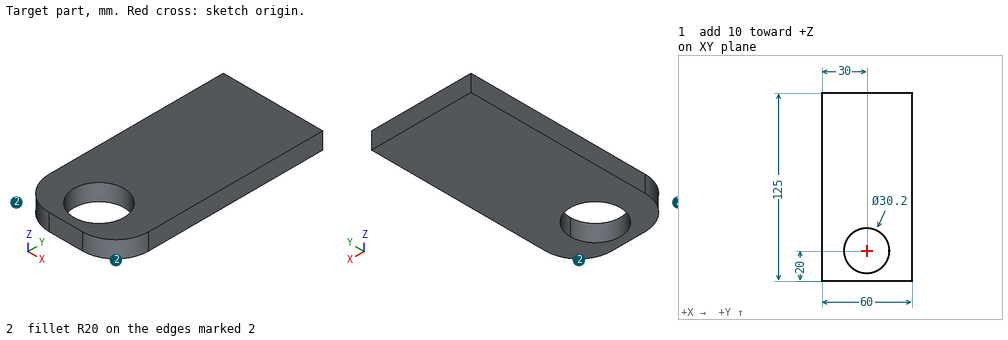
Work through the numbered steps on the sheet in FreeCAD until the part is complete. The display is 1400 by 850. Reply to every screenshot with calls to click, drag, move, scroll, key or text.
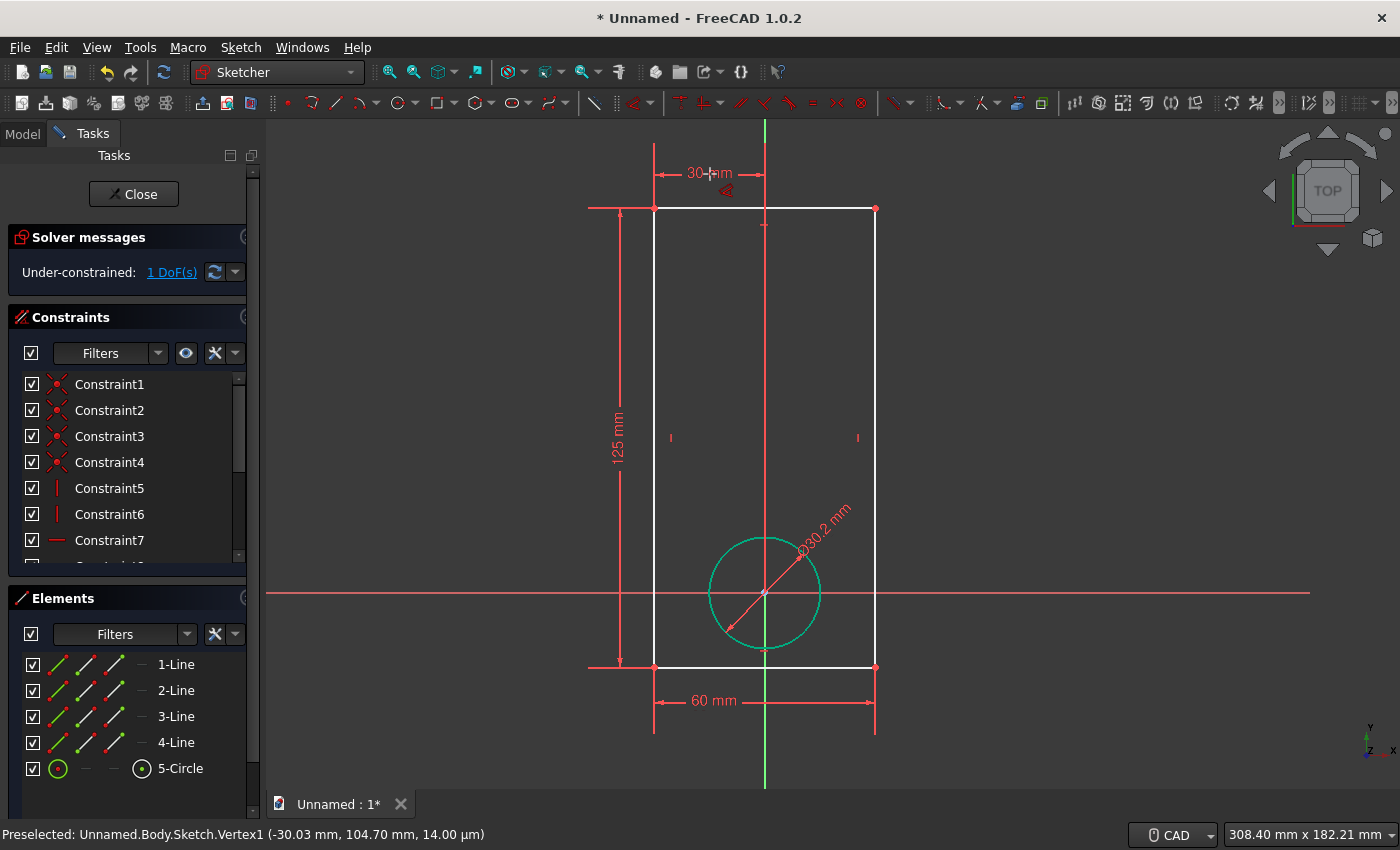
click(654, 668)
click(620, 630)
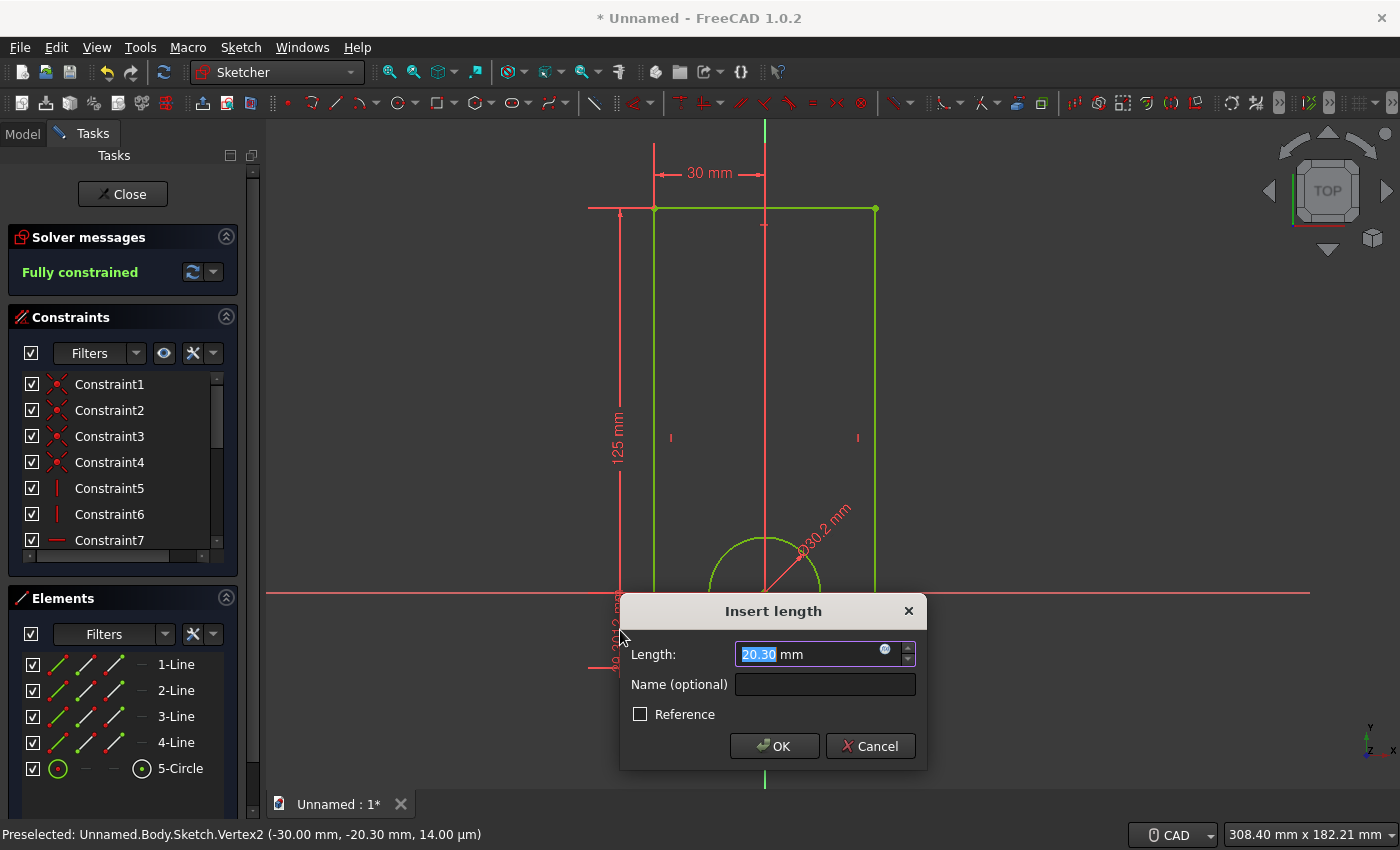
text(20)
key(Return)
key(Escape)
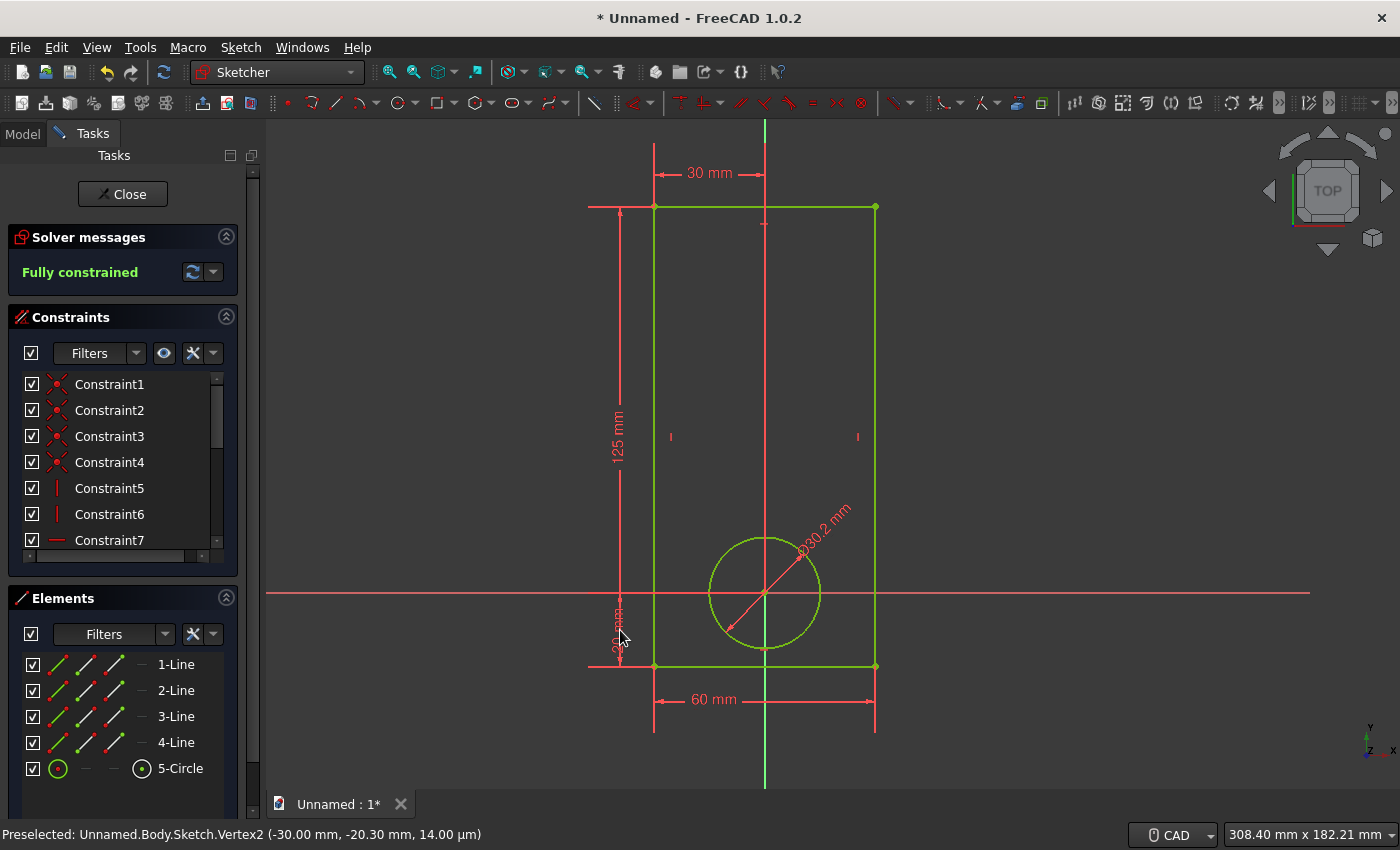
click(123, 194)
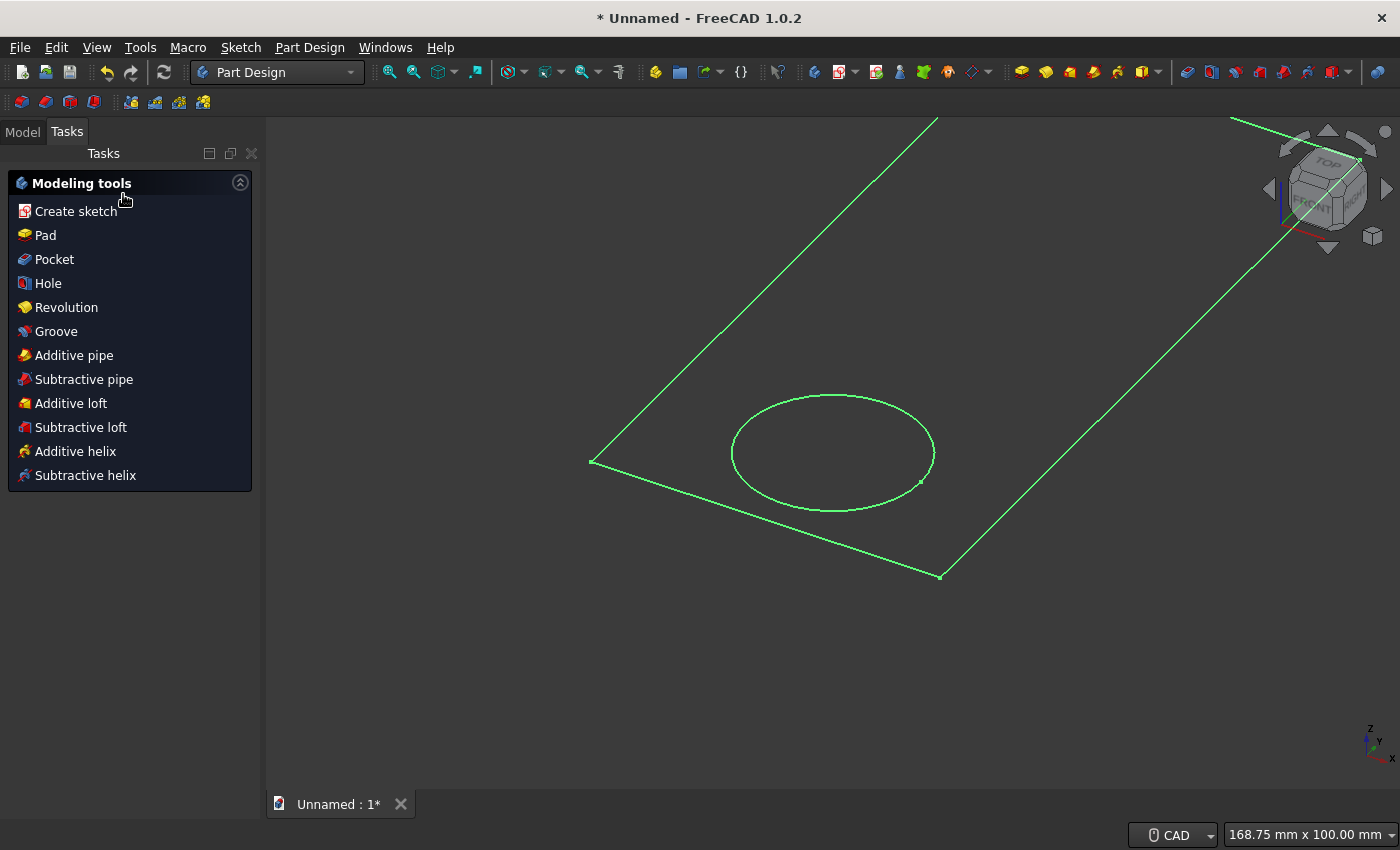
click(1022, 72)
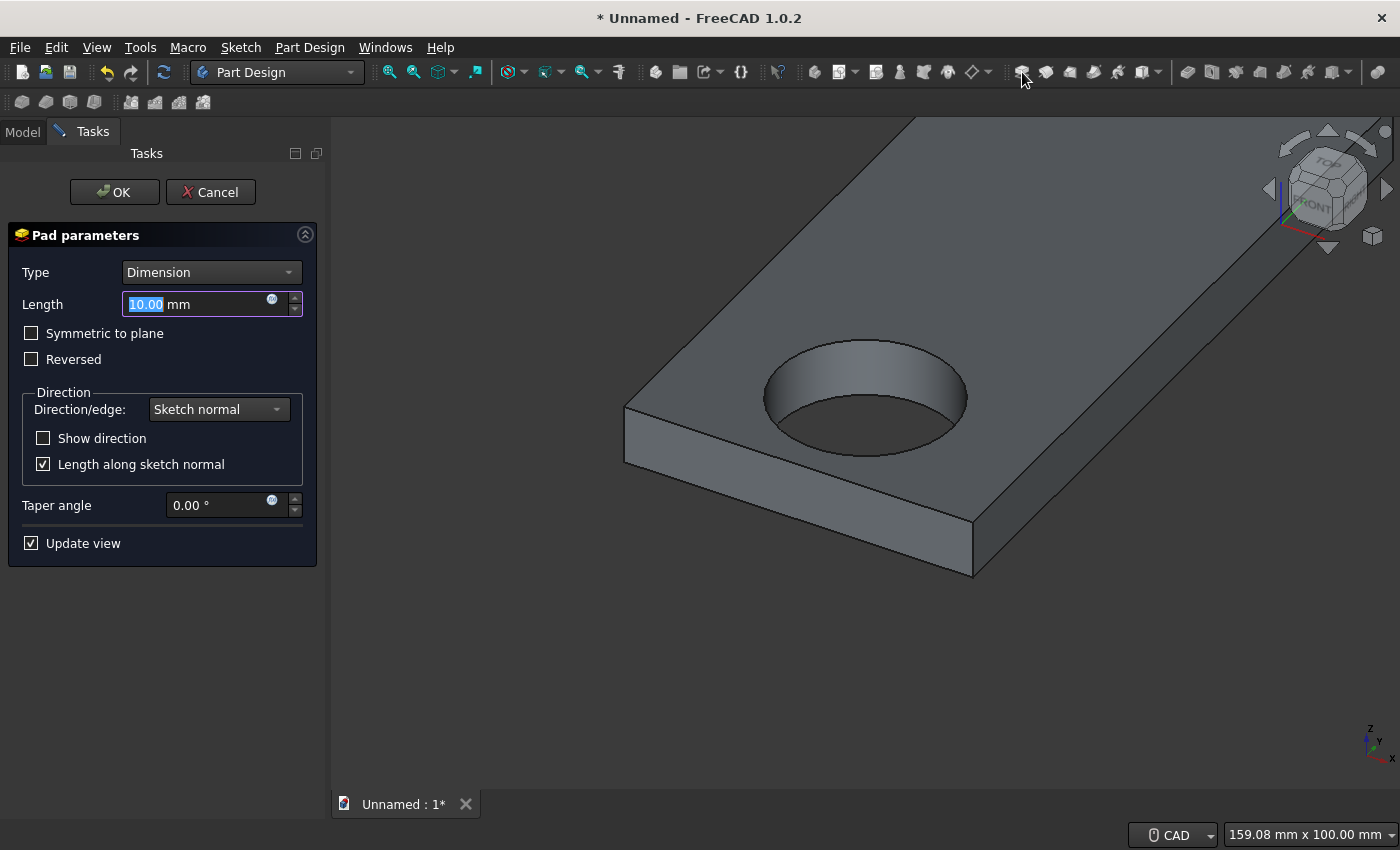
text(10)
key(Tab)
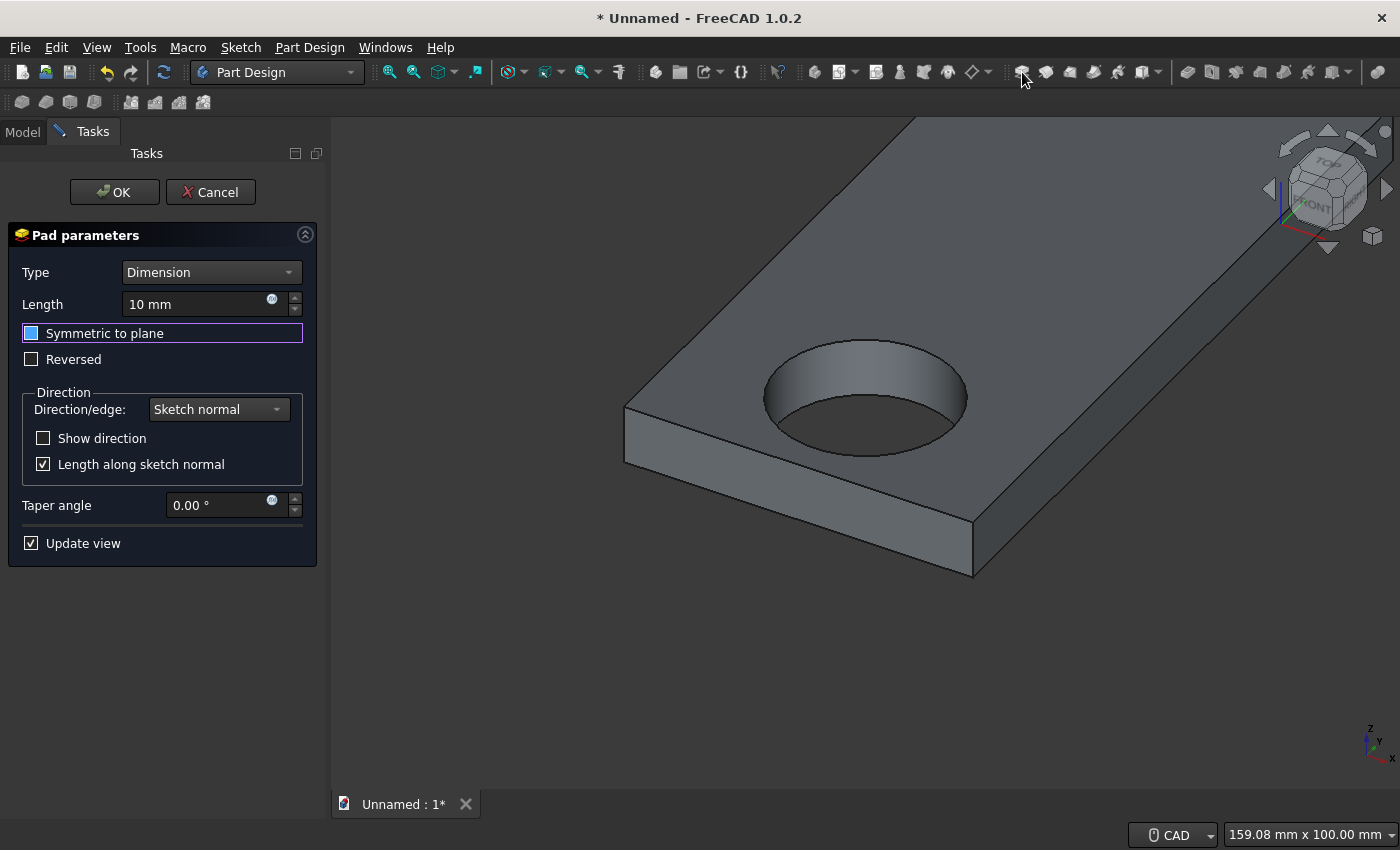
click(115, 192)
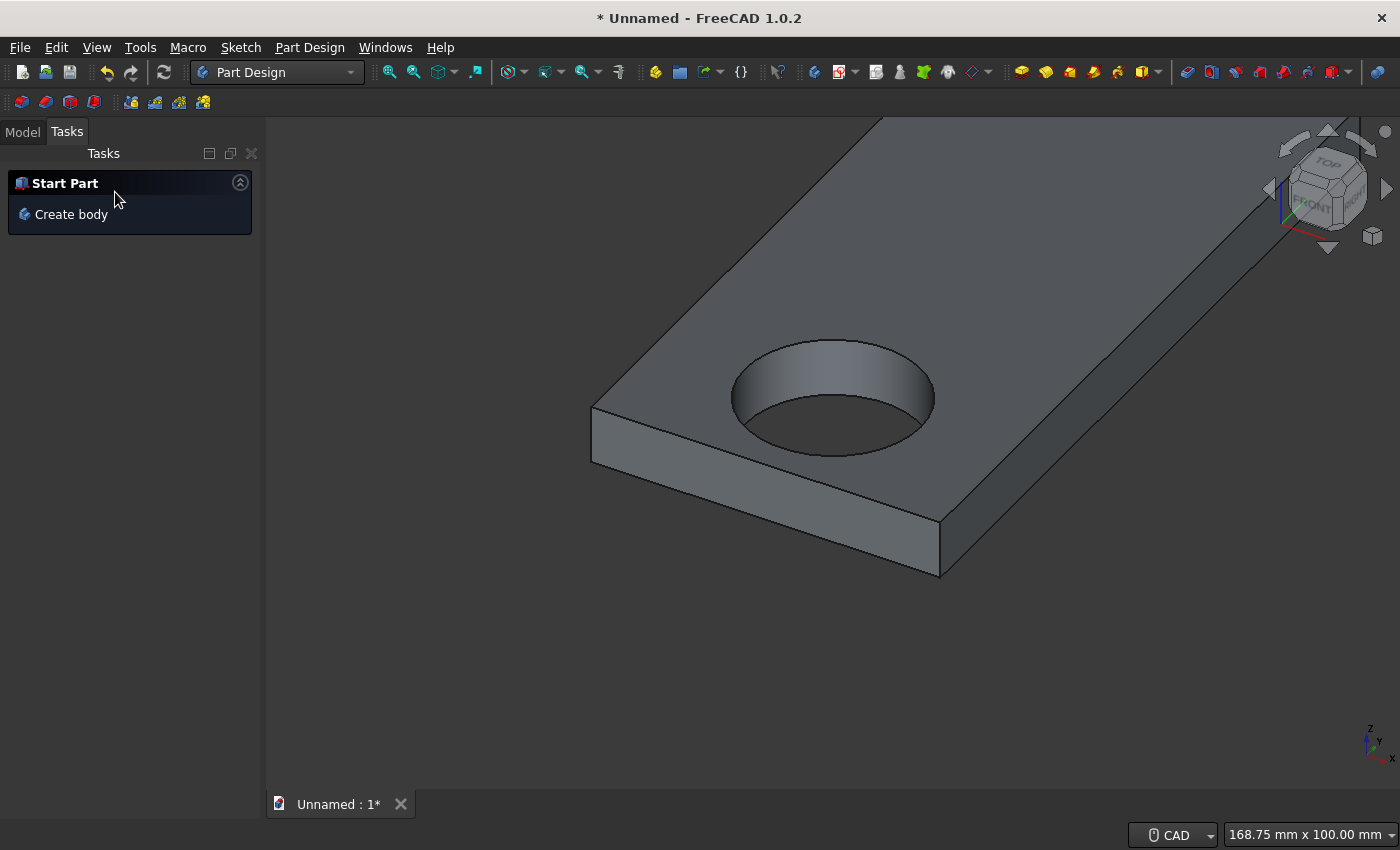
click(390, 72)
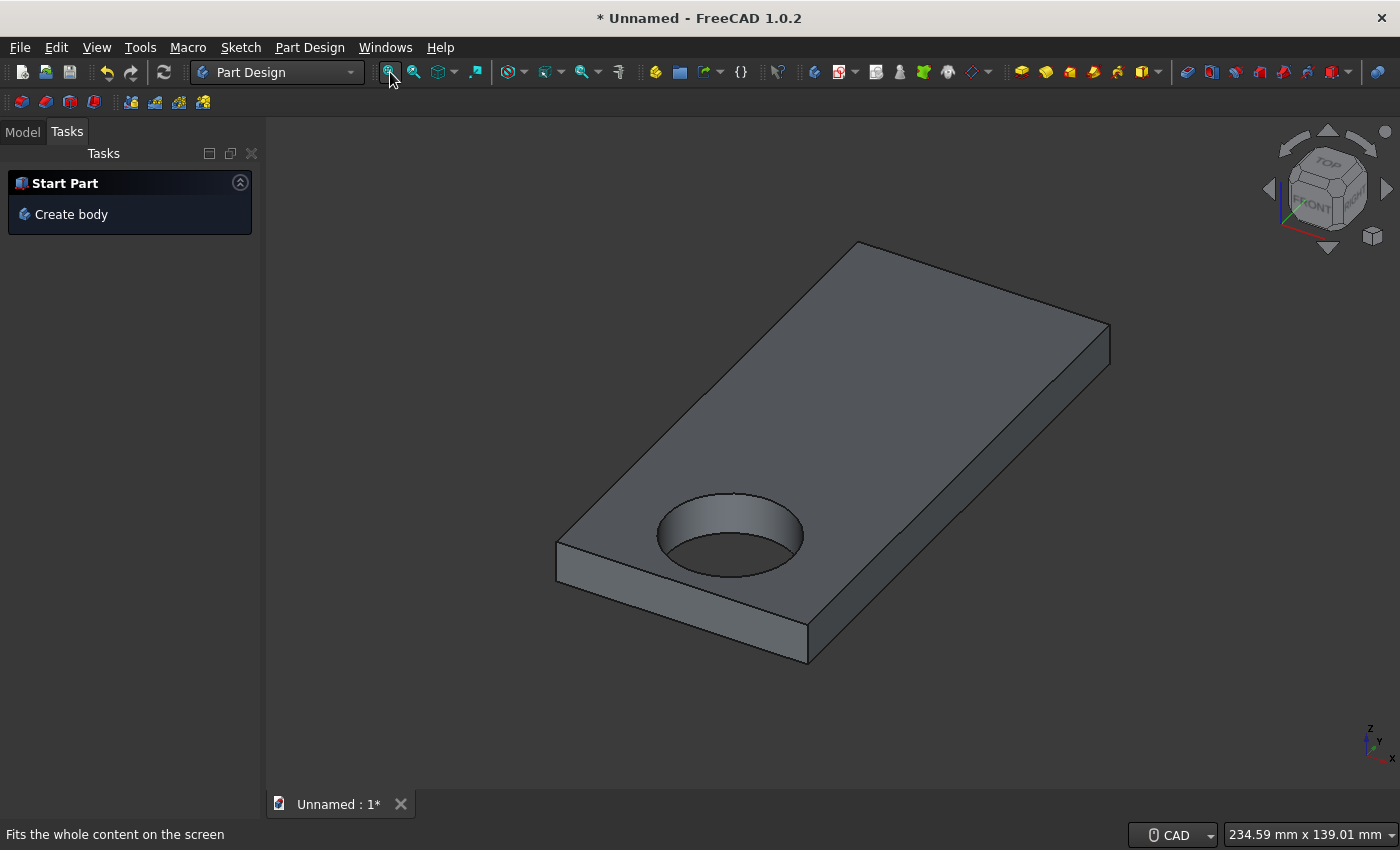
click(808, 644)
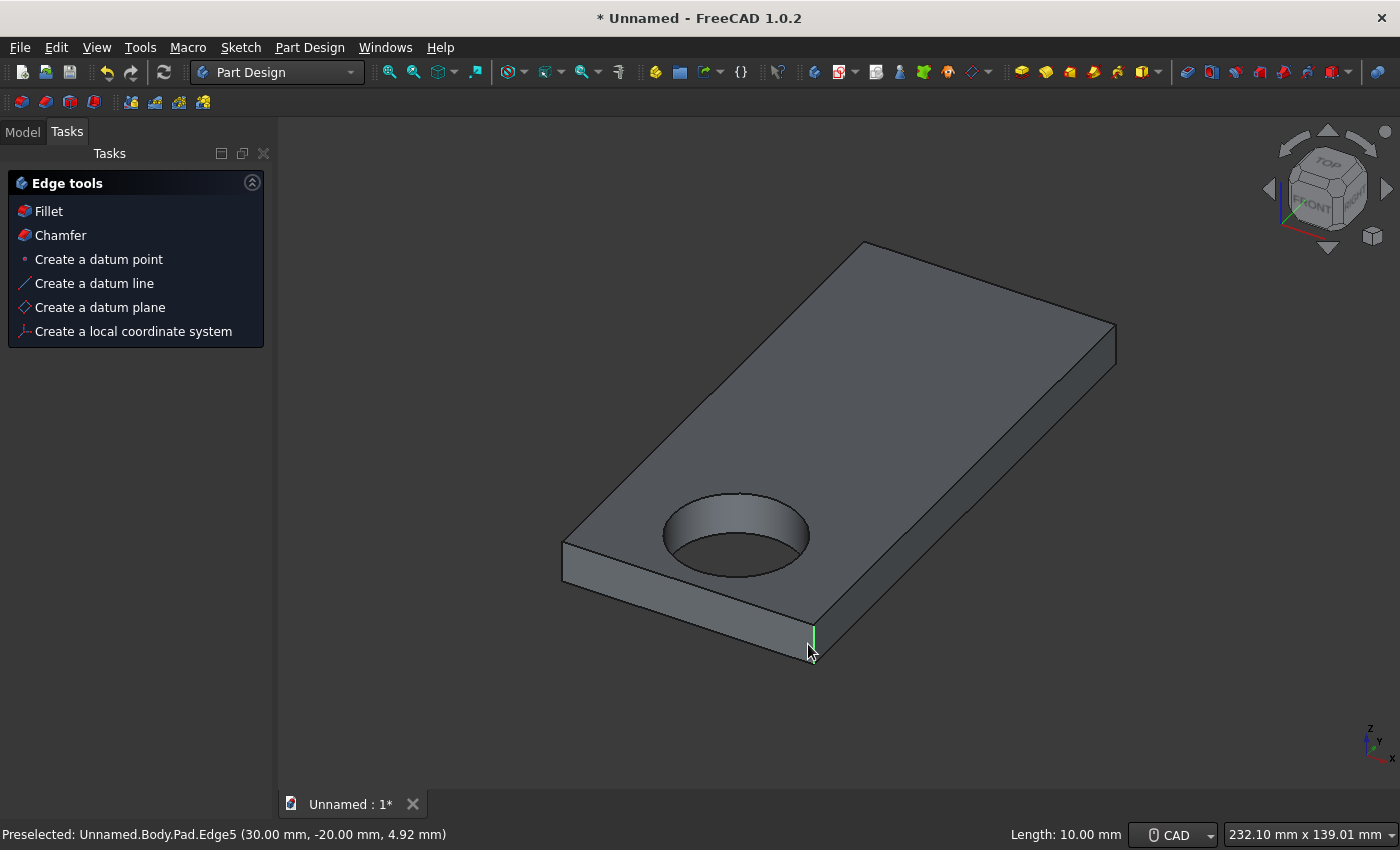
key(0)